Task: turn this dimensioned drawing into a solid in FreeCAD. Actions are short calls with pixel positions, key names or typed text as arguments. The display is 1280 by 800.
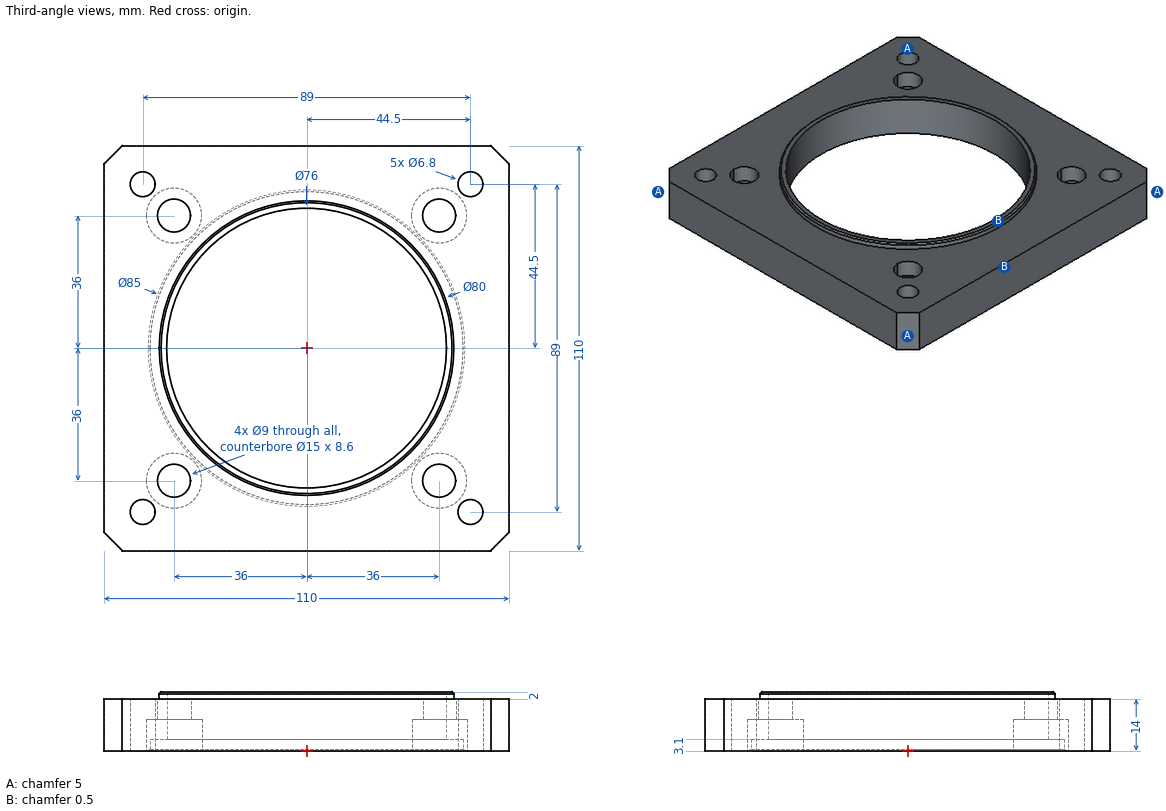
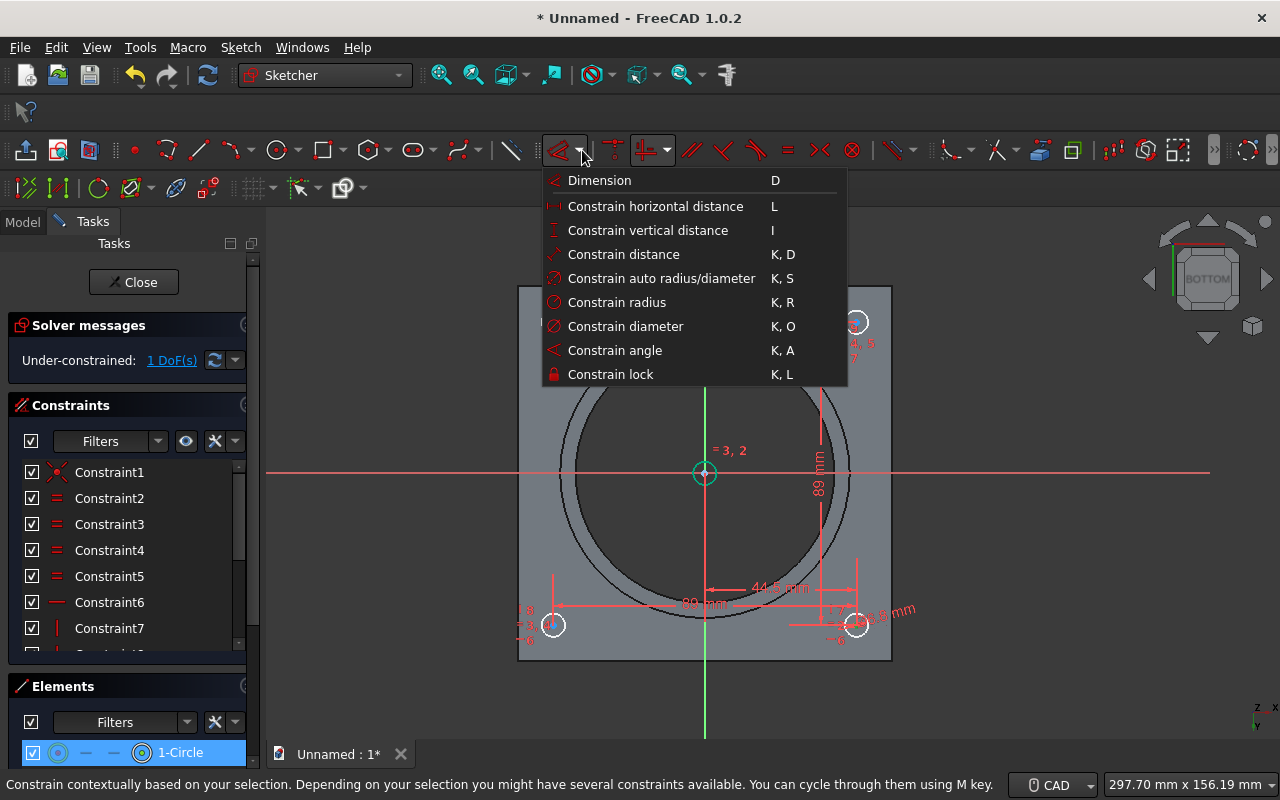
click(695, 230)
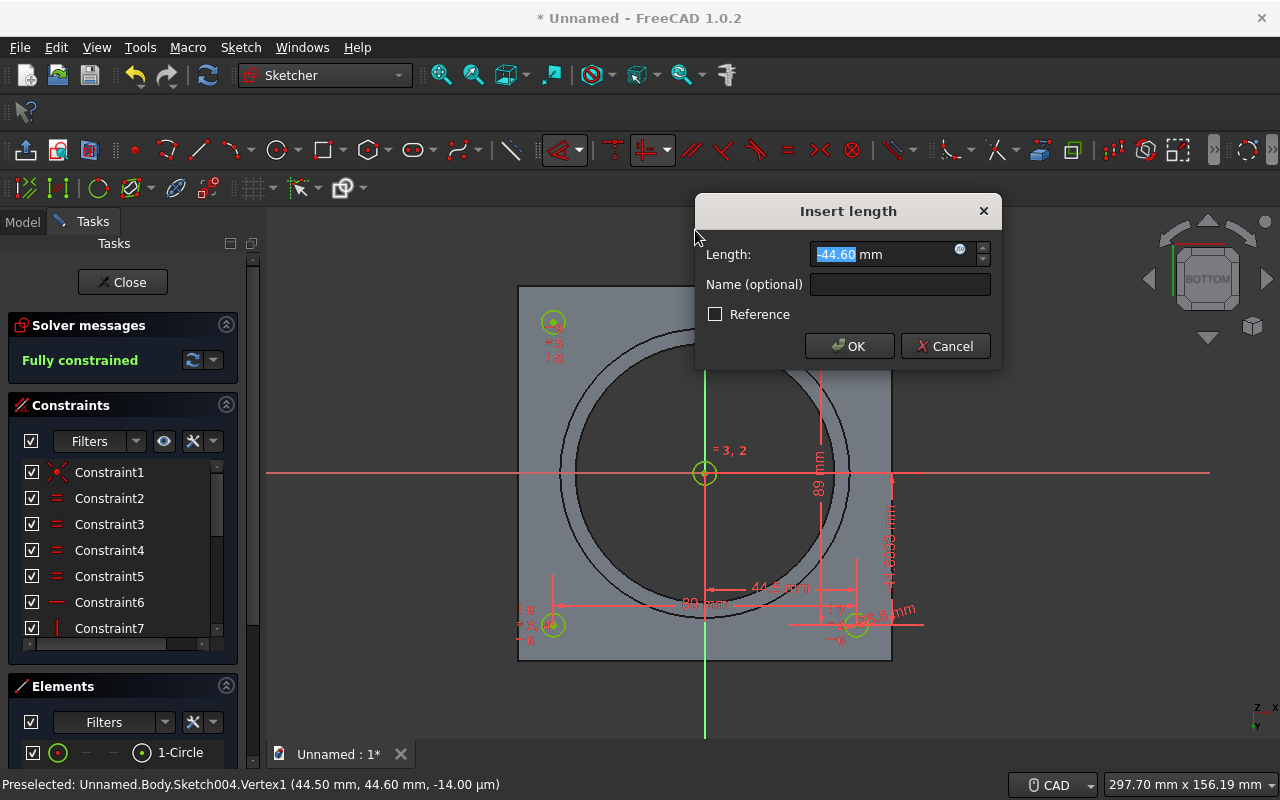
text(-44.5)
key(Return)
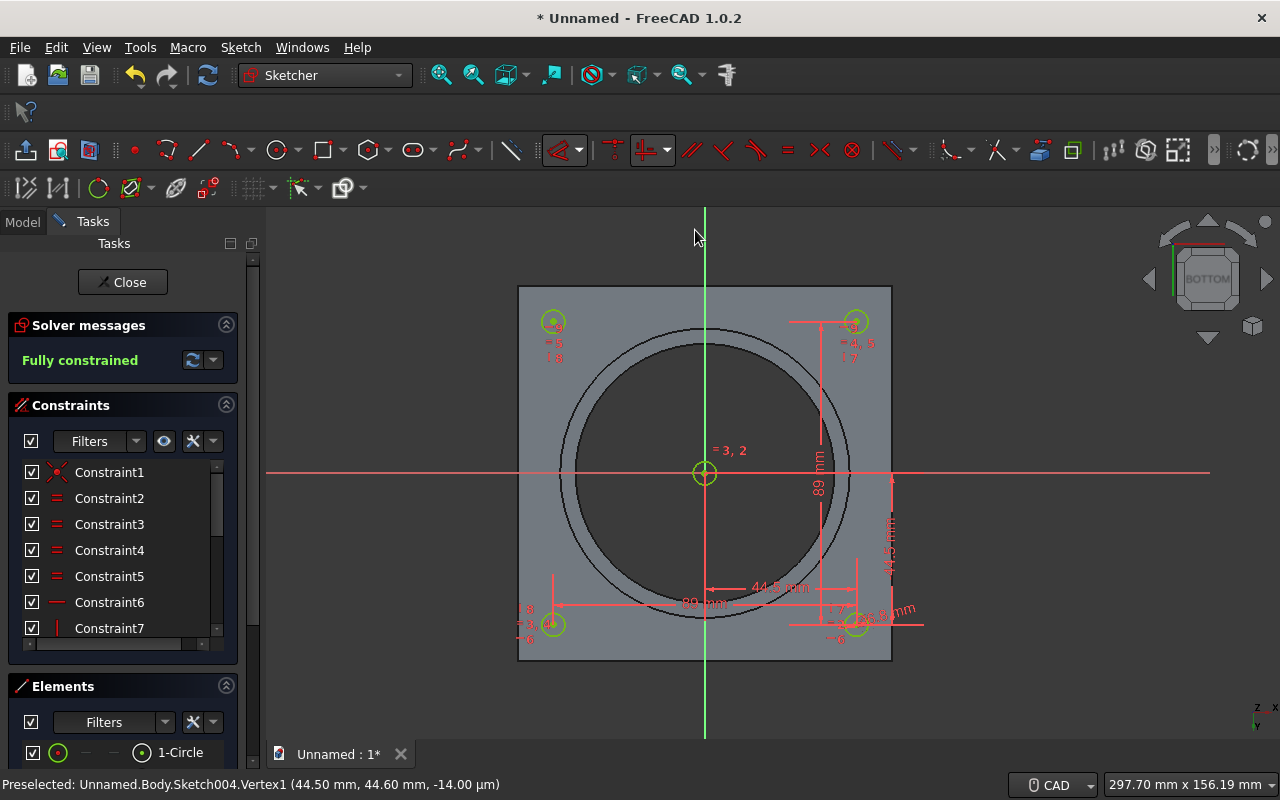
click(123, 282)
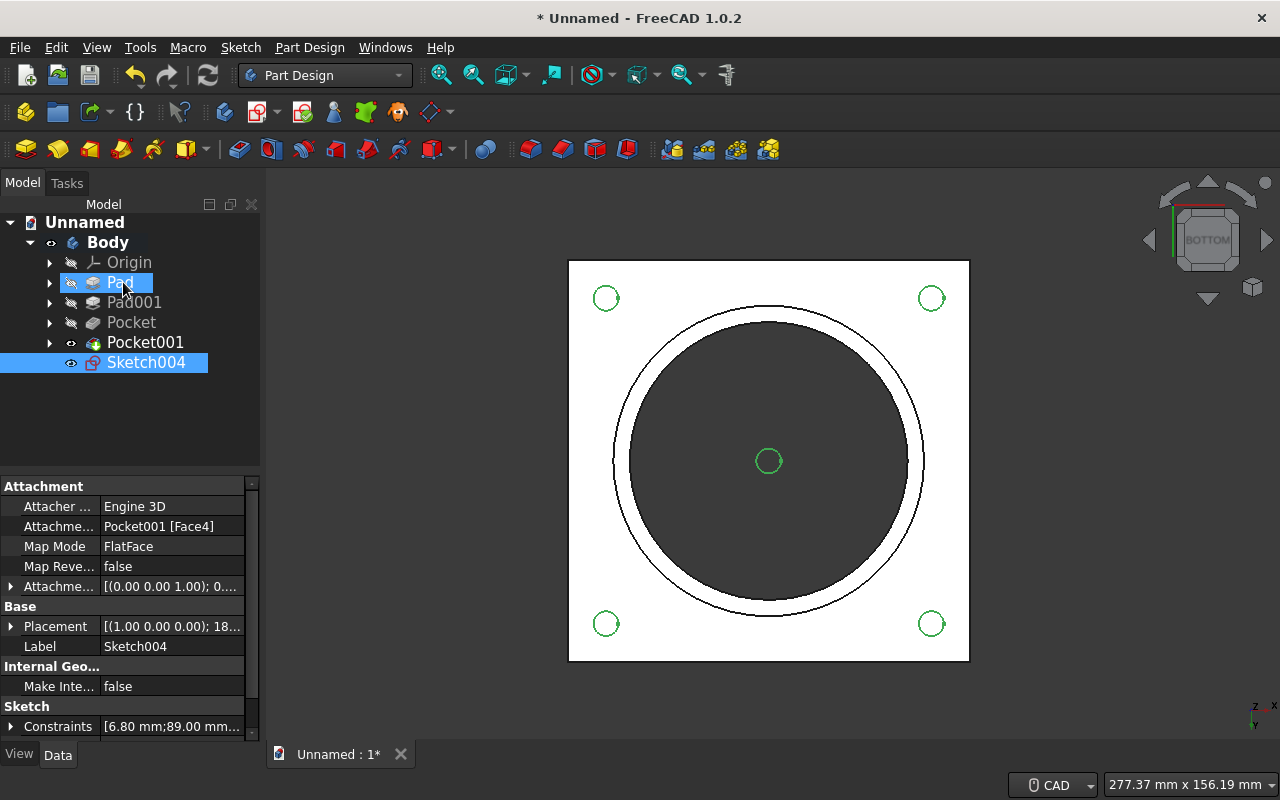
click(240, 150)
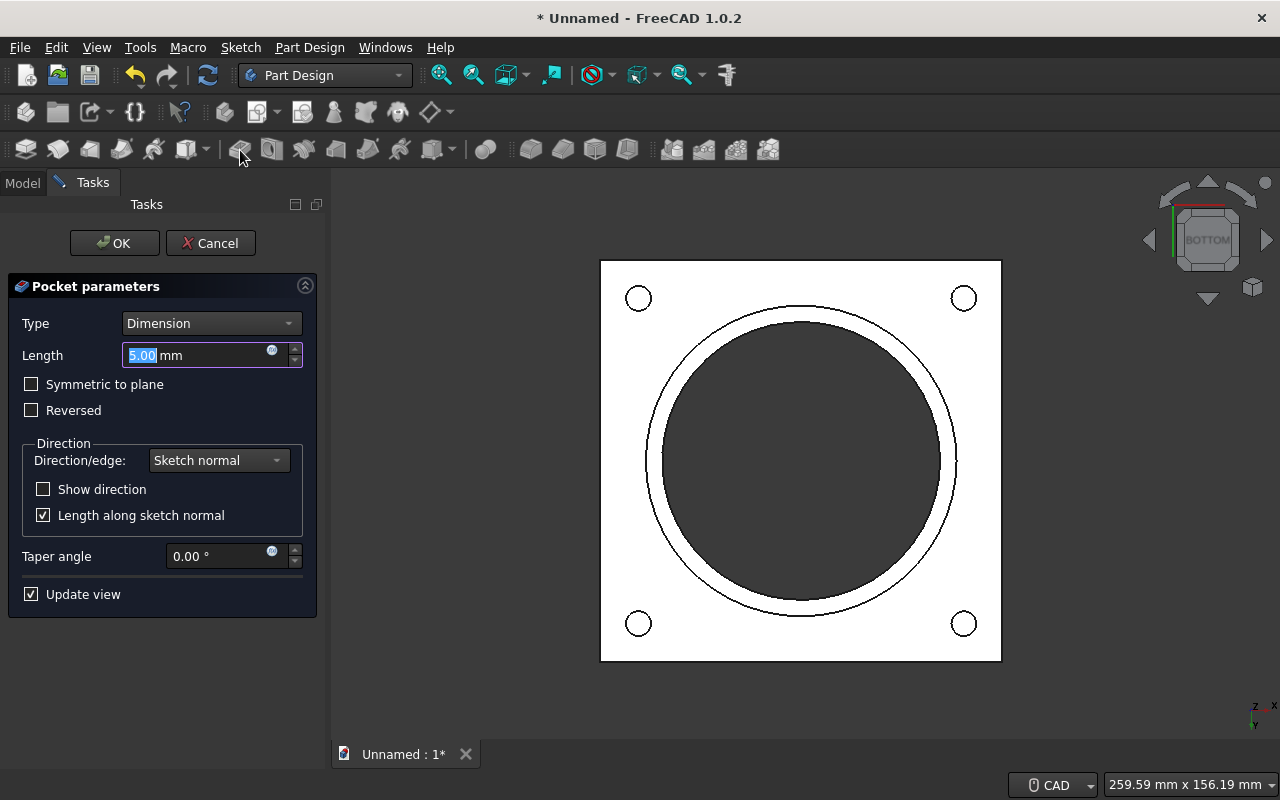
click(212, 324)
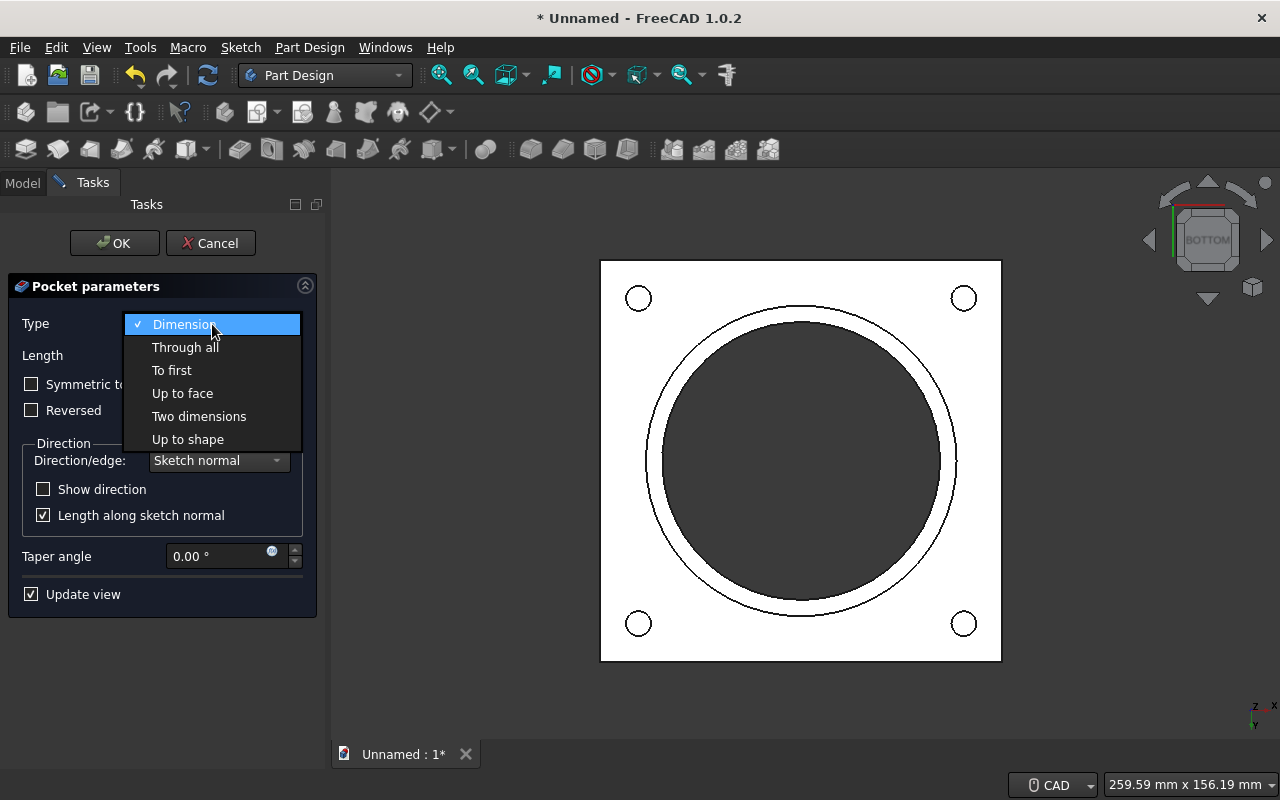
click(212, 348)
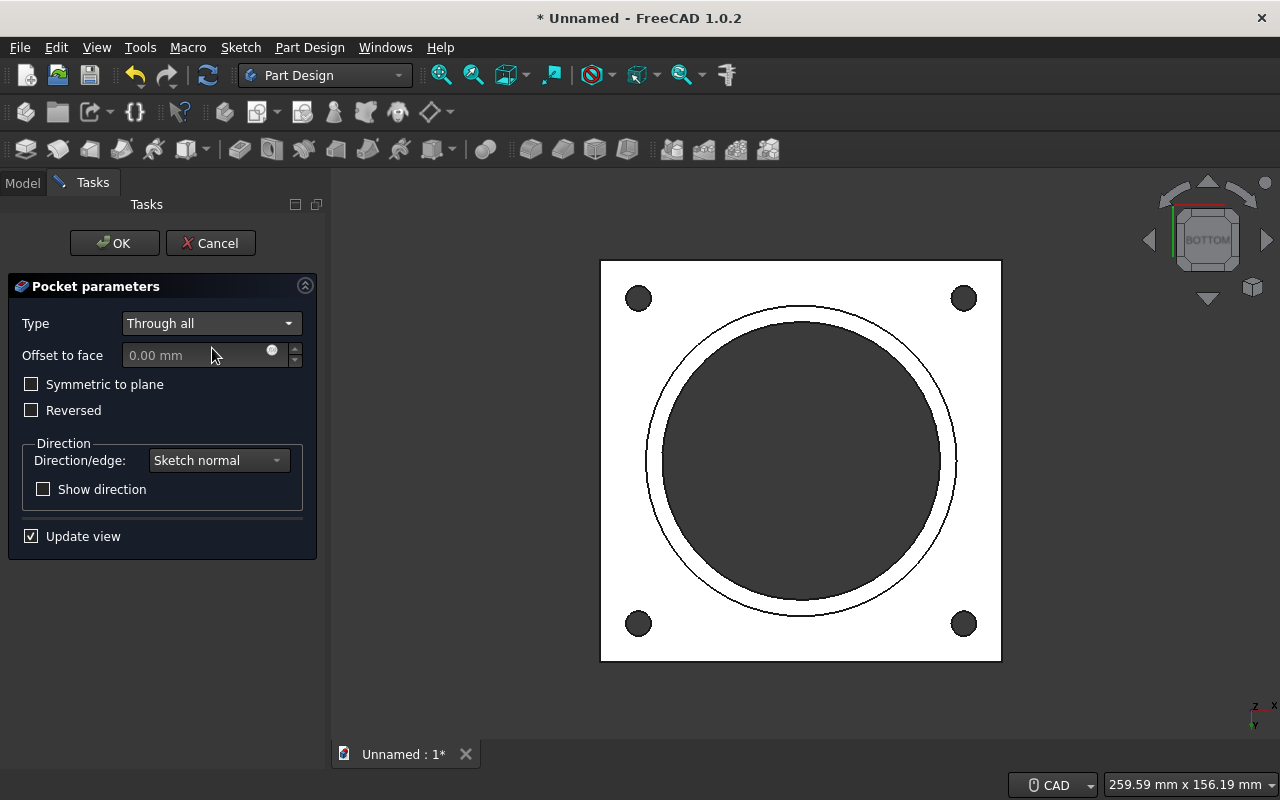
click(115, 243)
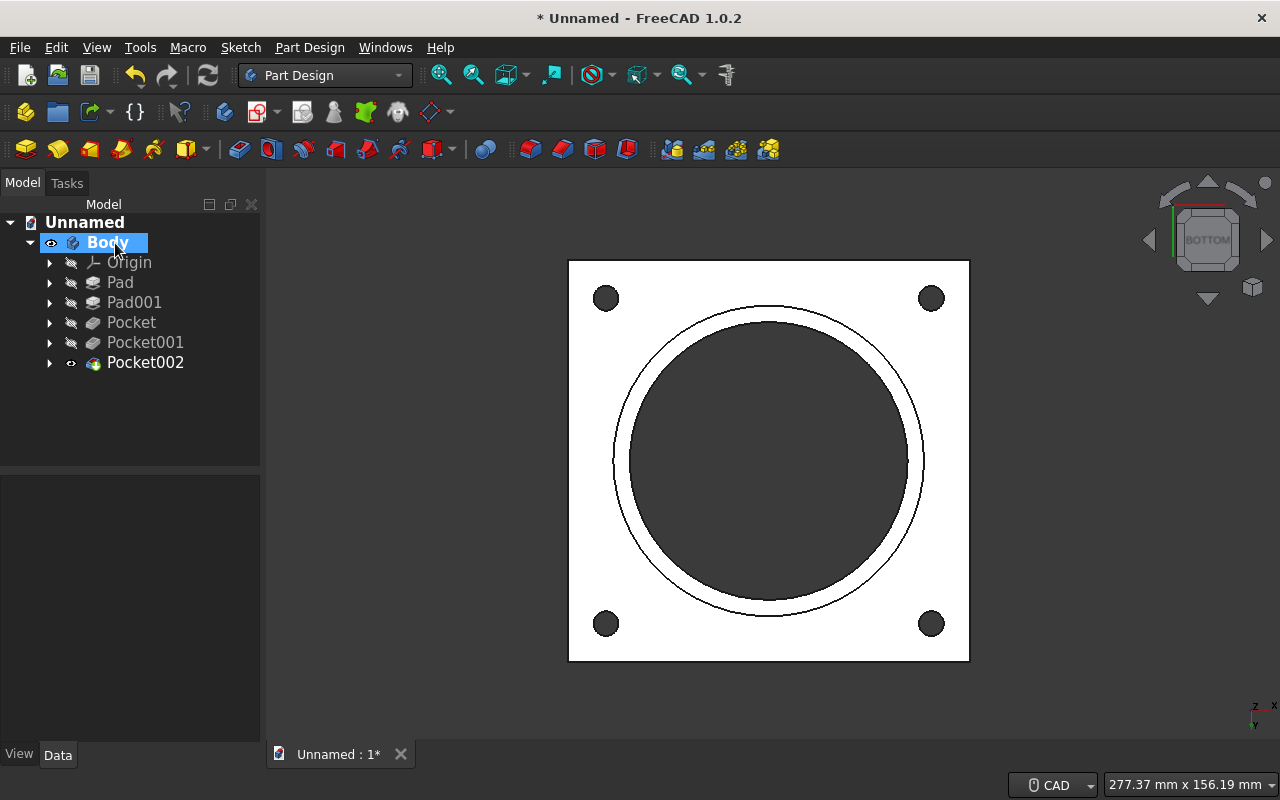
click(941, 575)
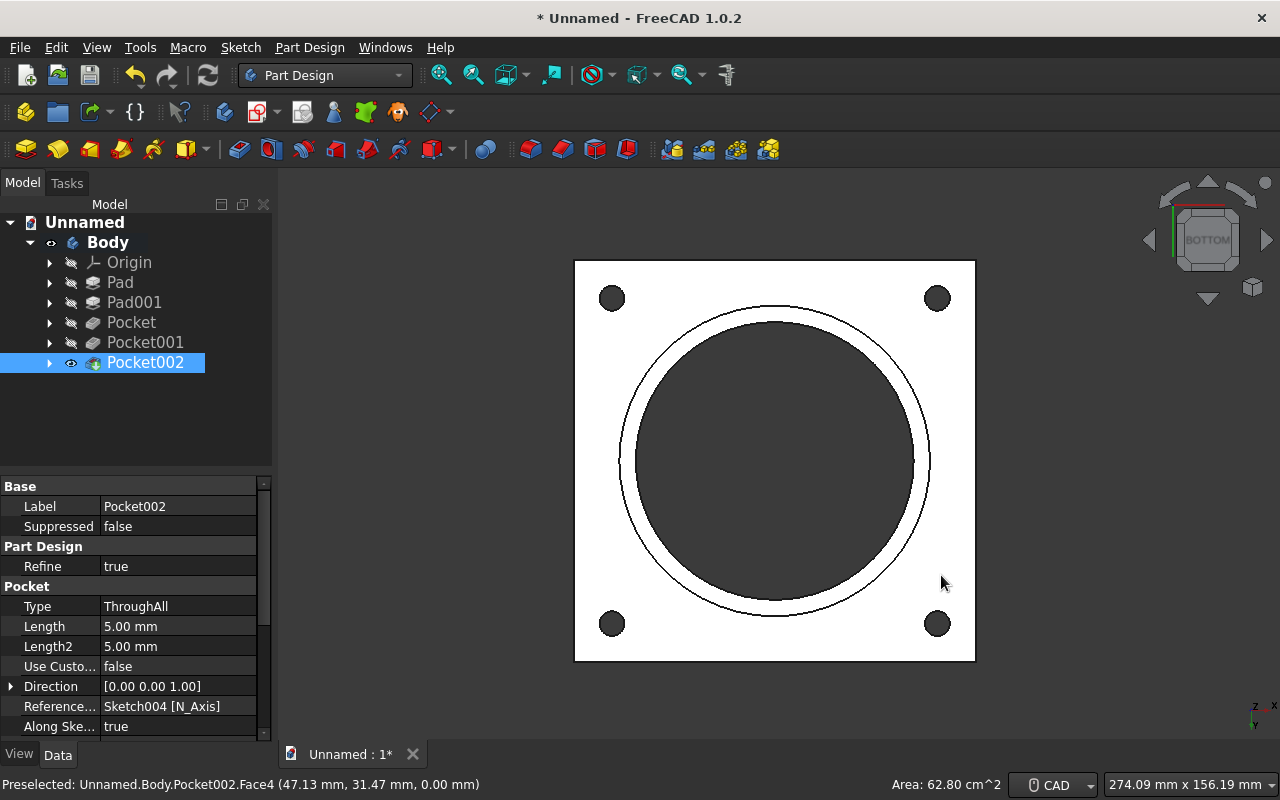
click(258, 112)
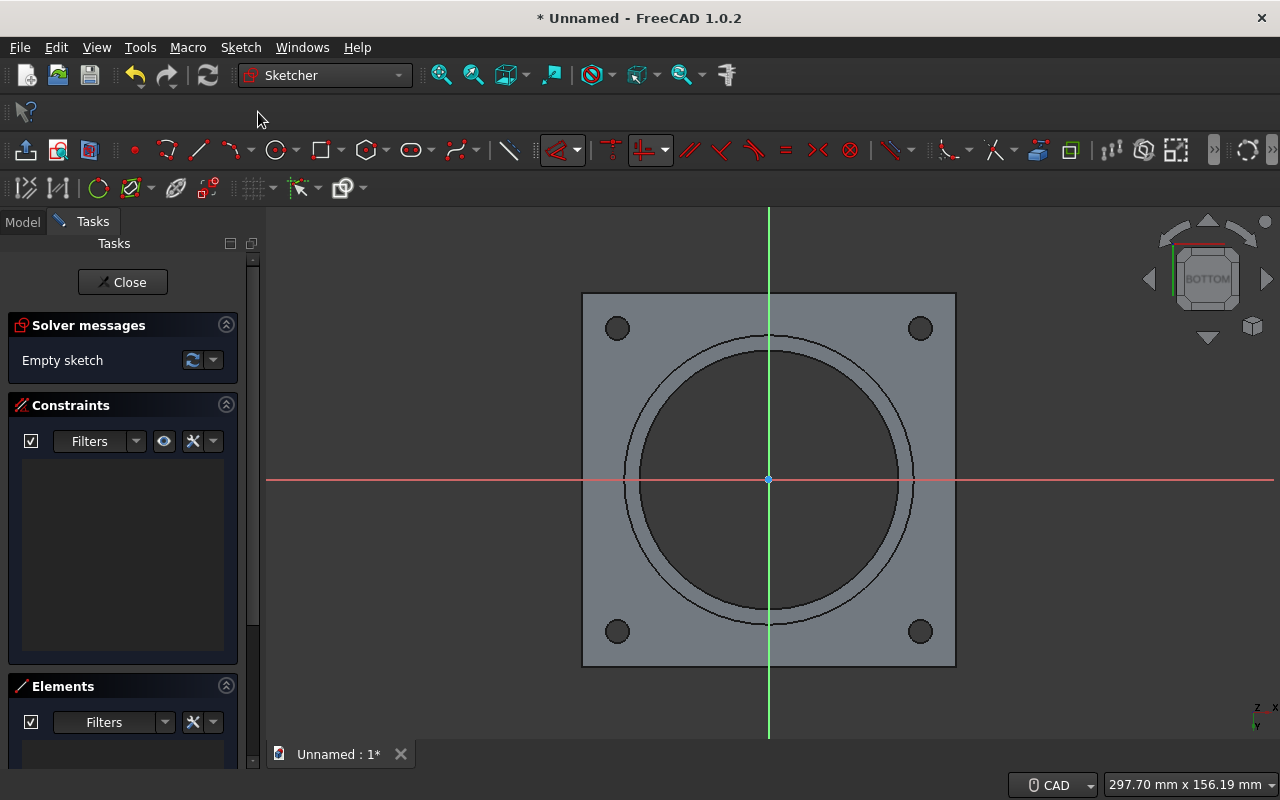
click(276, 150)